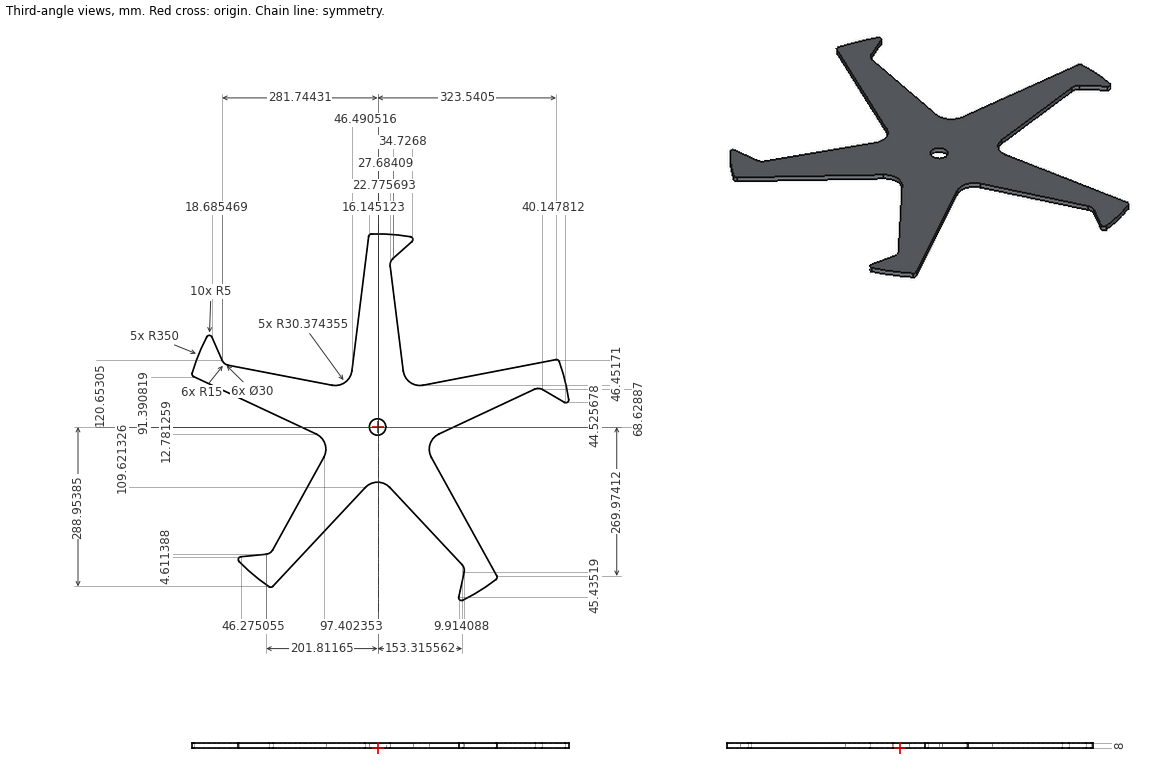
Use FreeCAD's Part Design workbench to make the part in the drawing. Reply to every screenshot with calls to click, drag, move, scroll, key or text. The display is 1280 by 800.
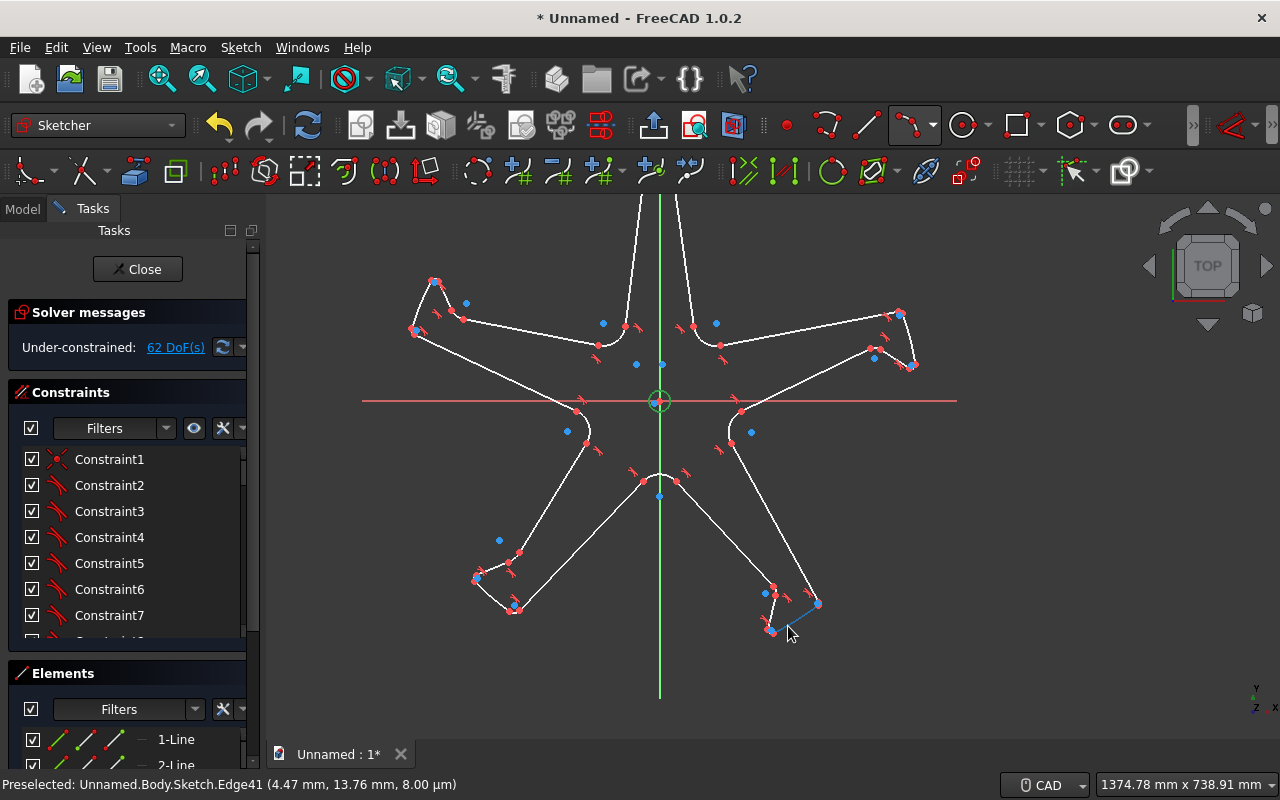
click(787, 626)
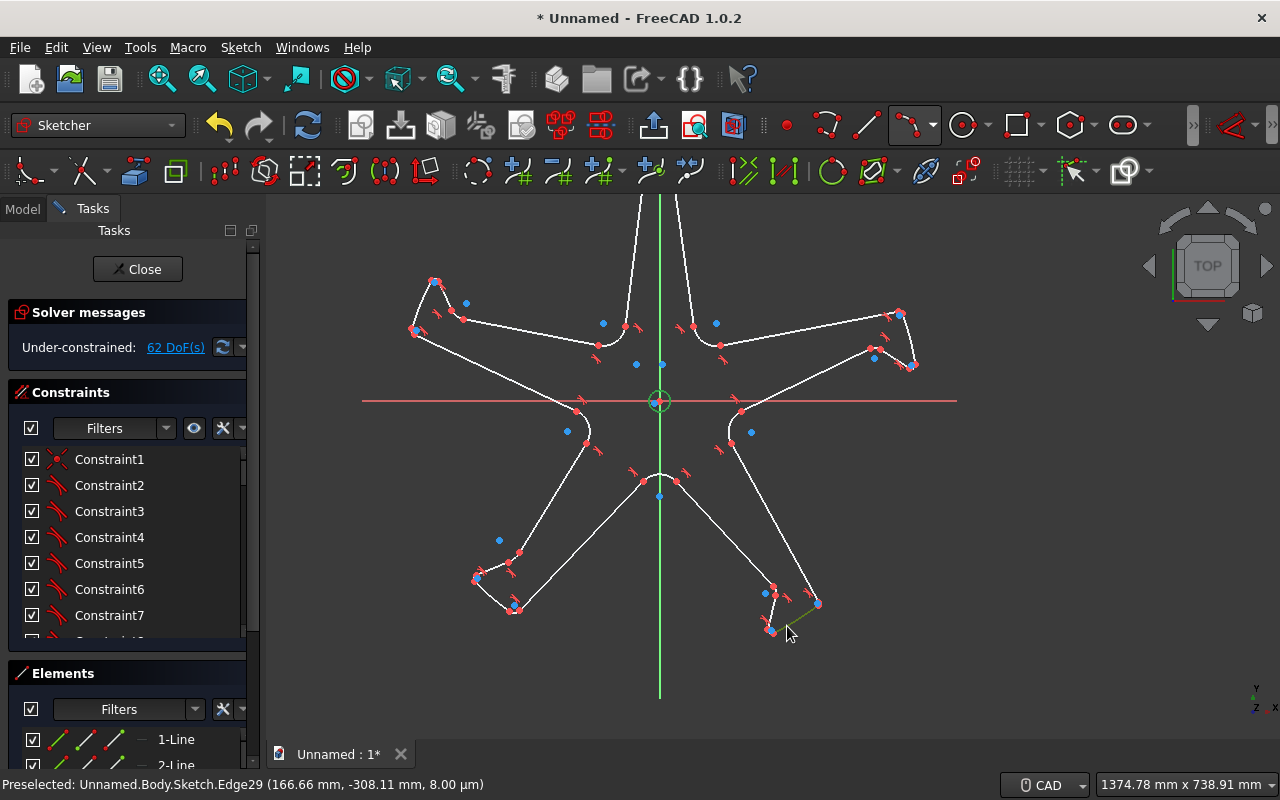
key(c)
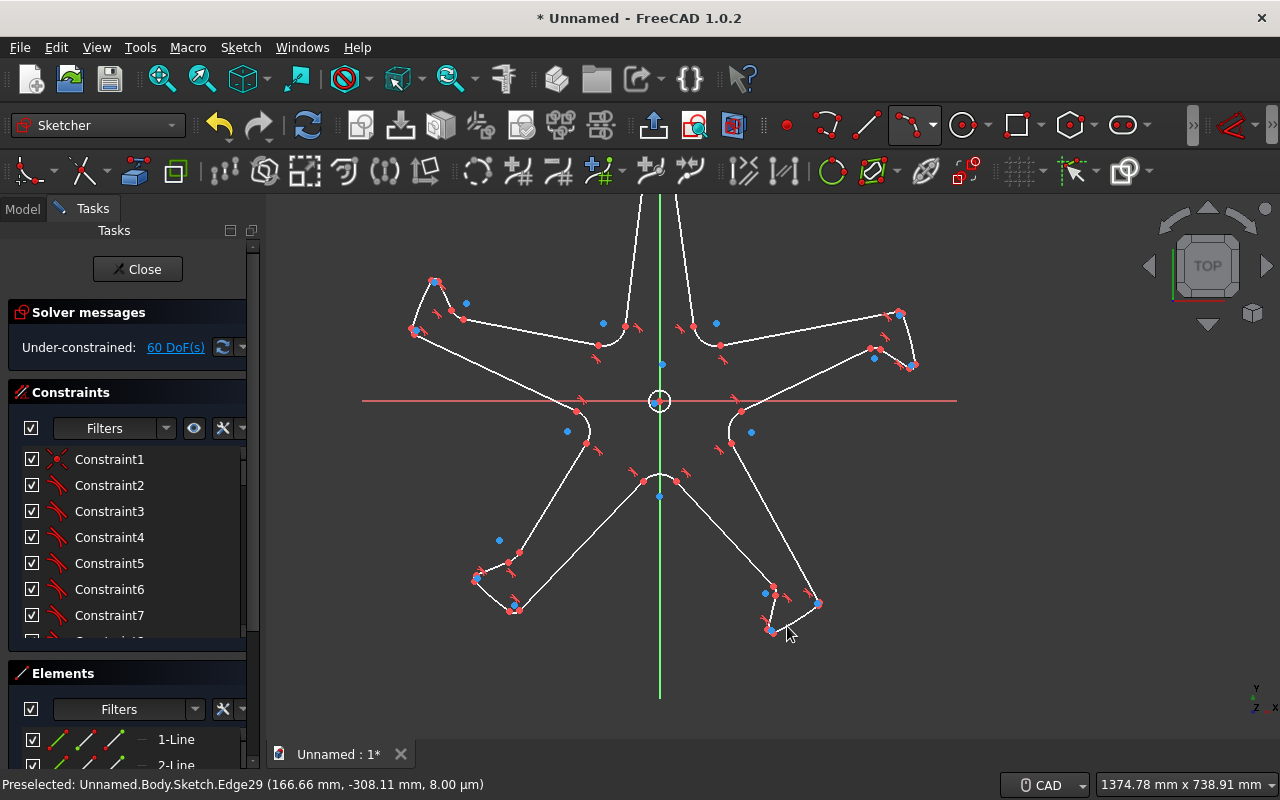
scroll(660, 391, up, 2)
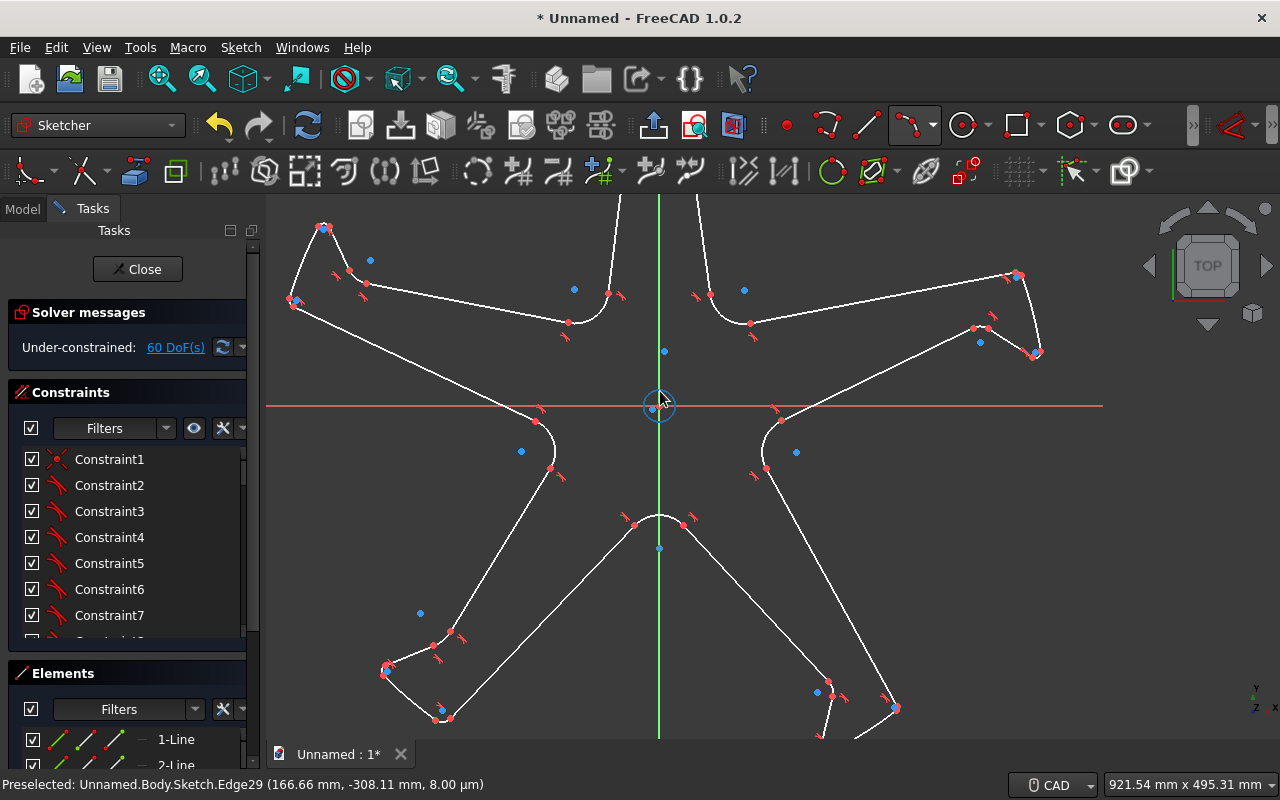
click(660, 390)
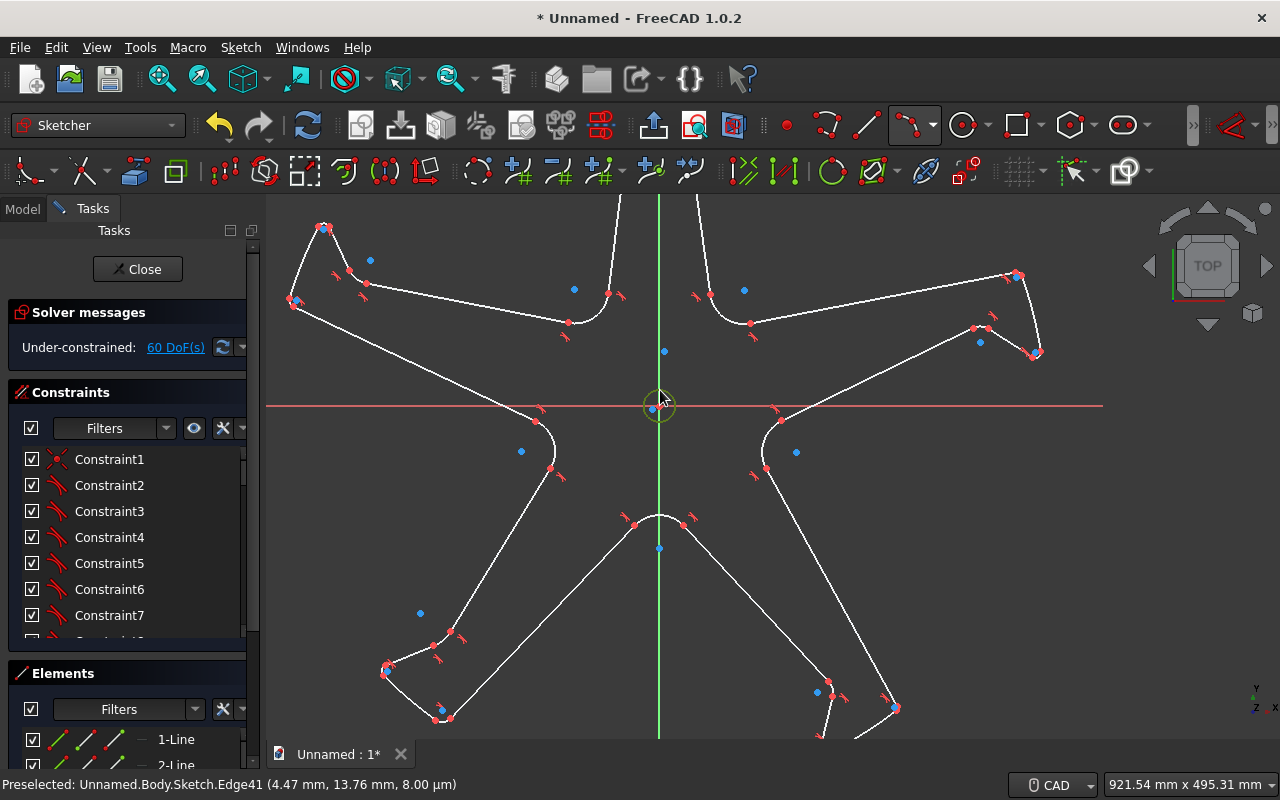
click(1037, 329)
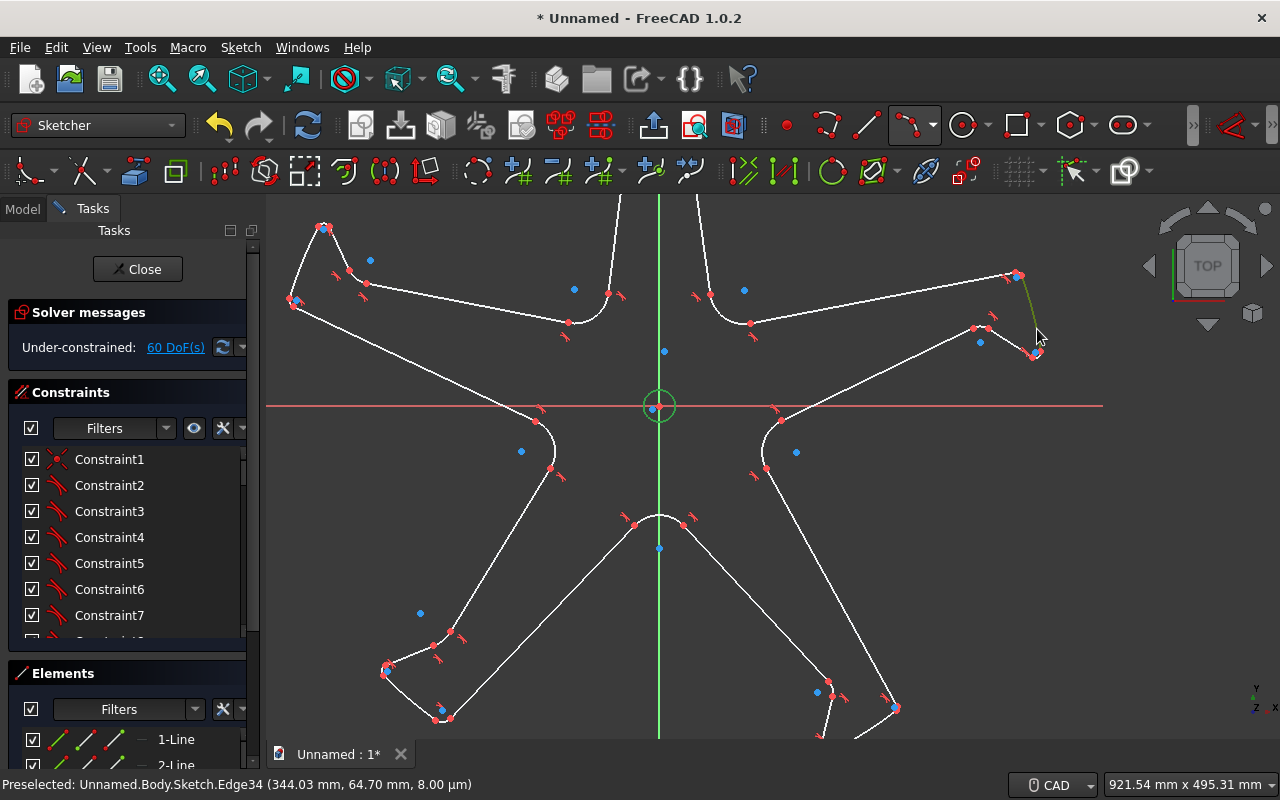
key(c)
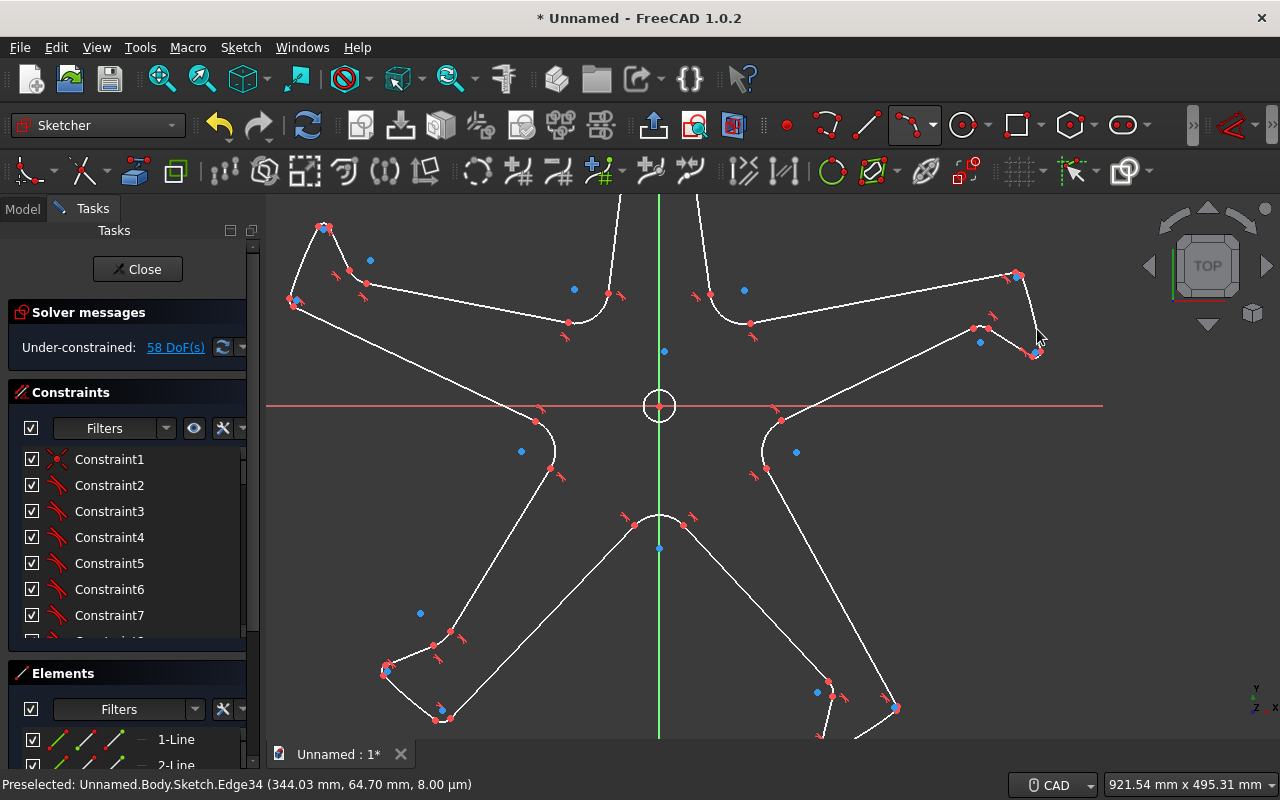
scroll(671, 395, up, 2)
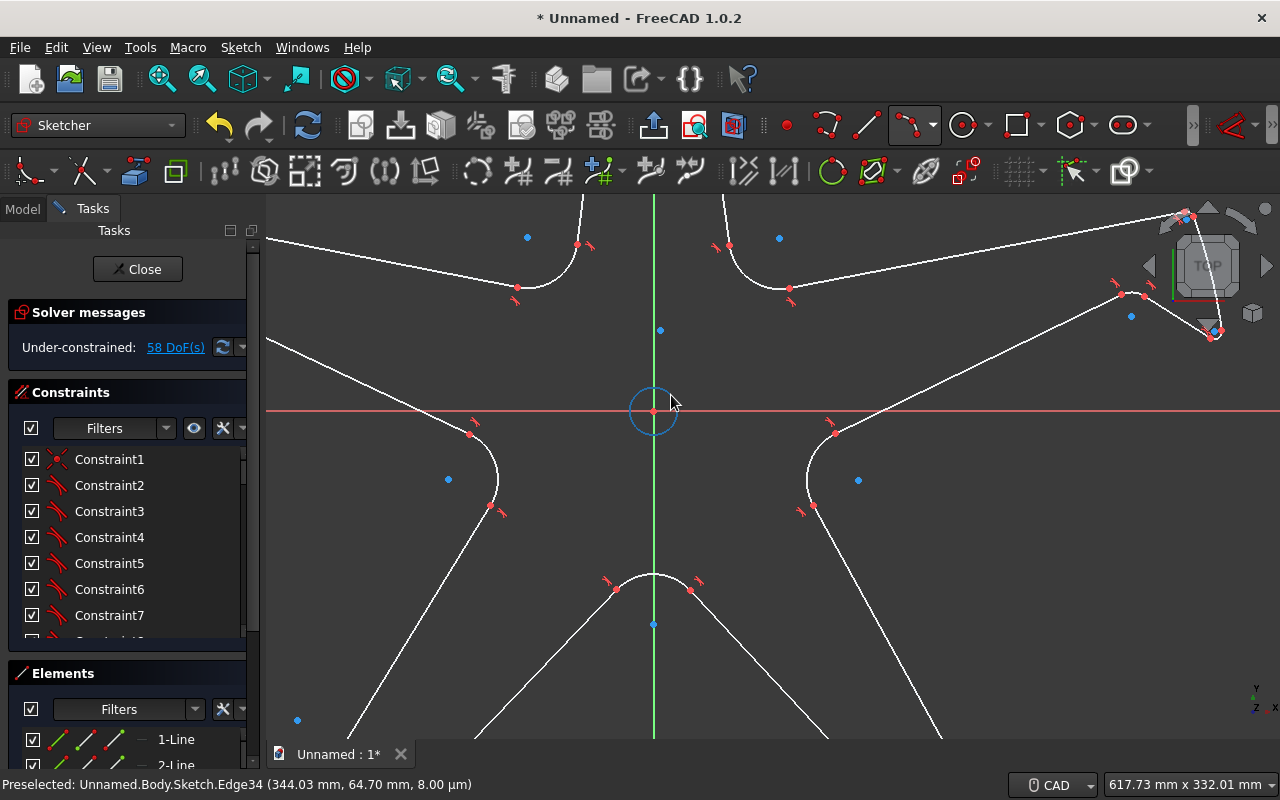
click(670, 394)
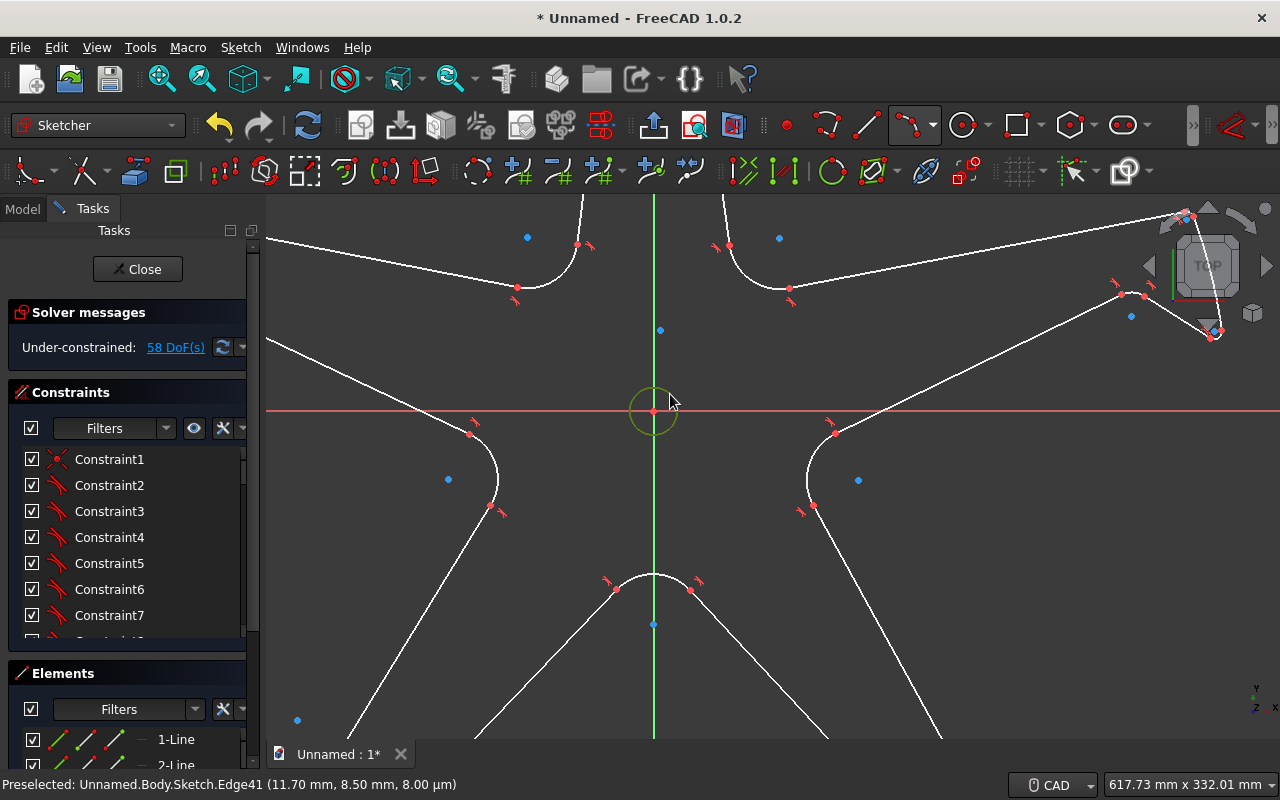
scroll(723, 503, down, 6)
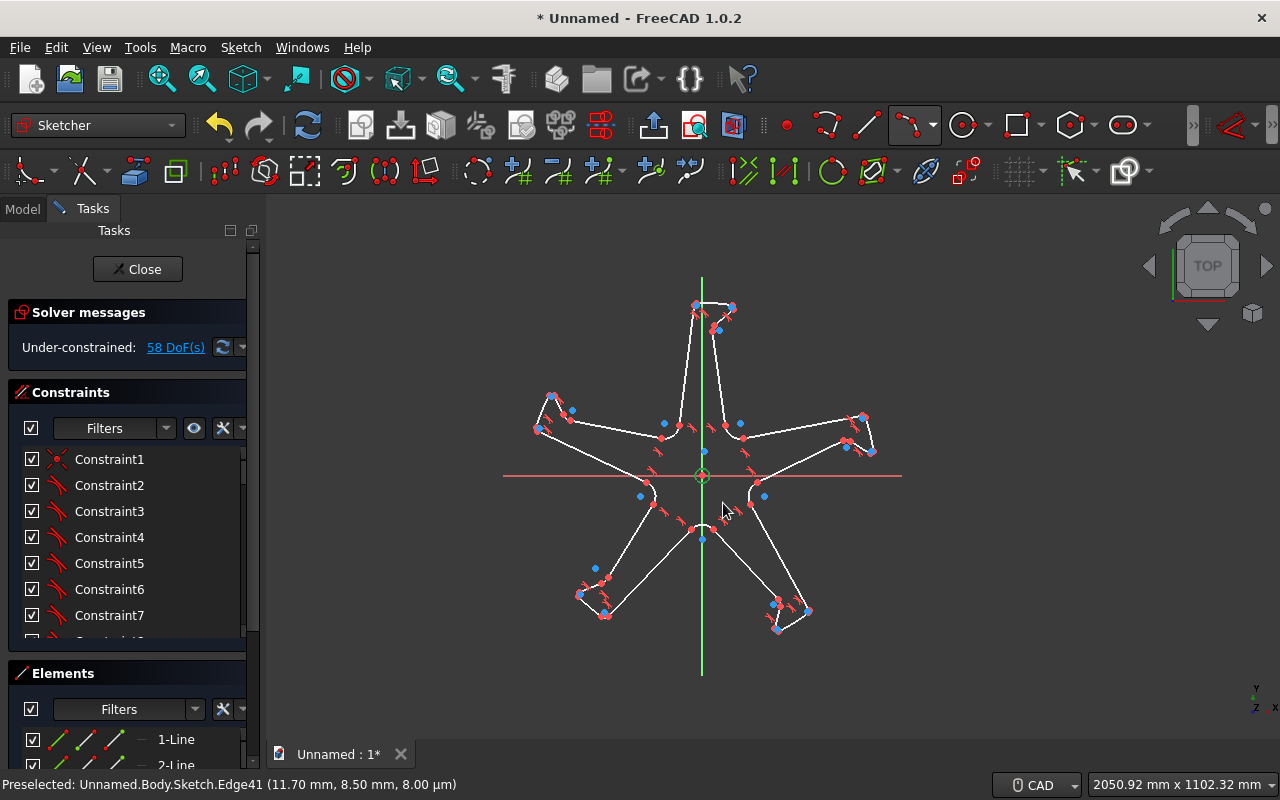
scroll(721, 304, up, 2)